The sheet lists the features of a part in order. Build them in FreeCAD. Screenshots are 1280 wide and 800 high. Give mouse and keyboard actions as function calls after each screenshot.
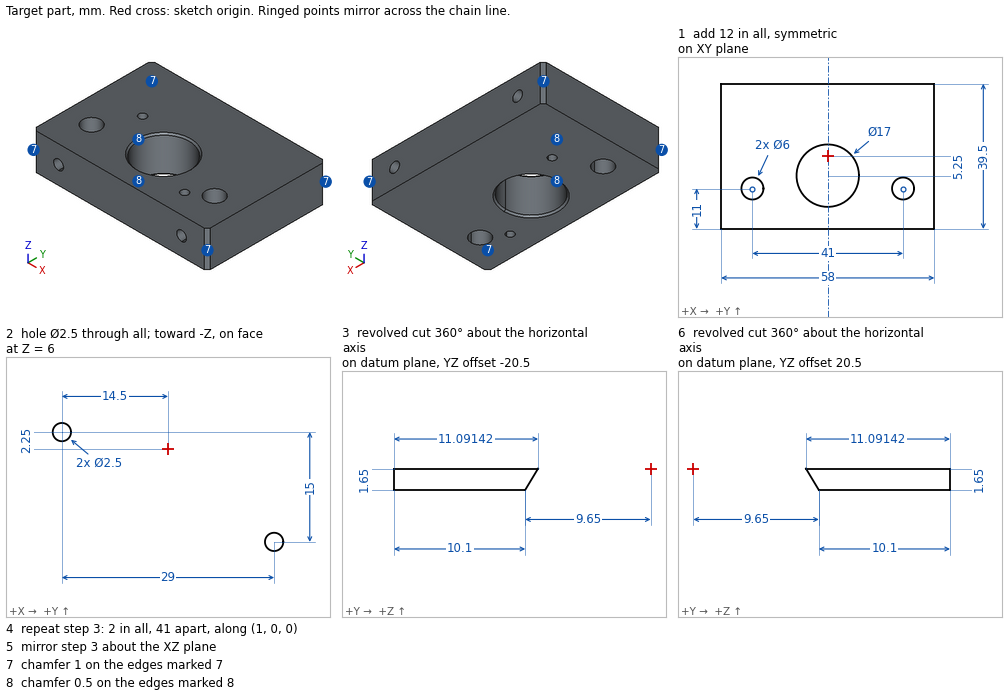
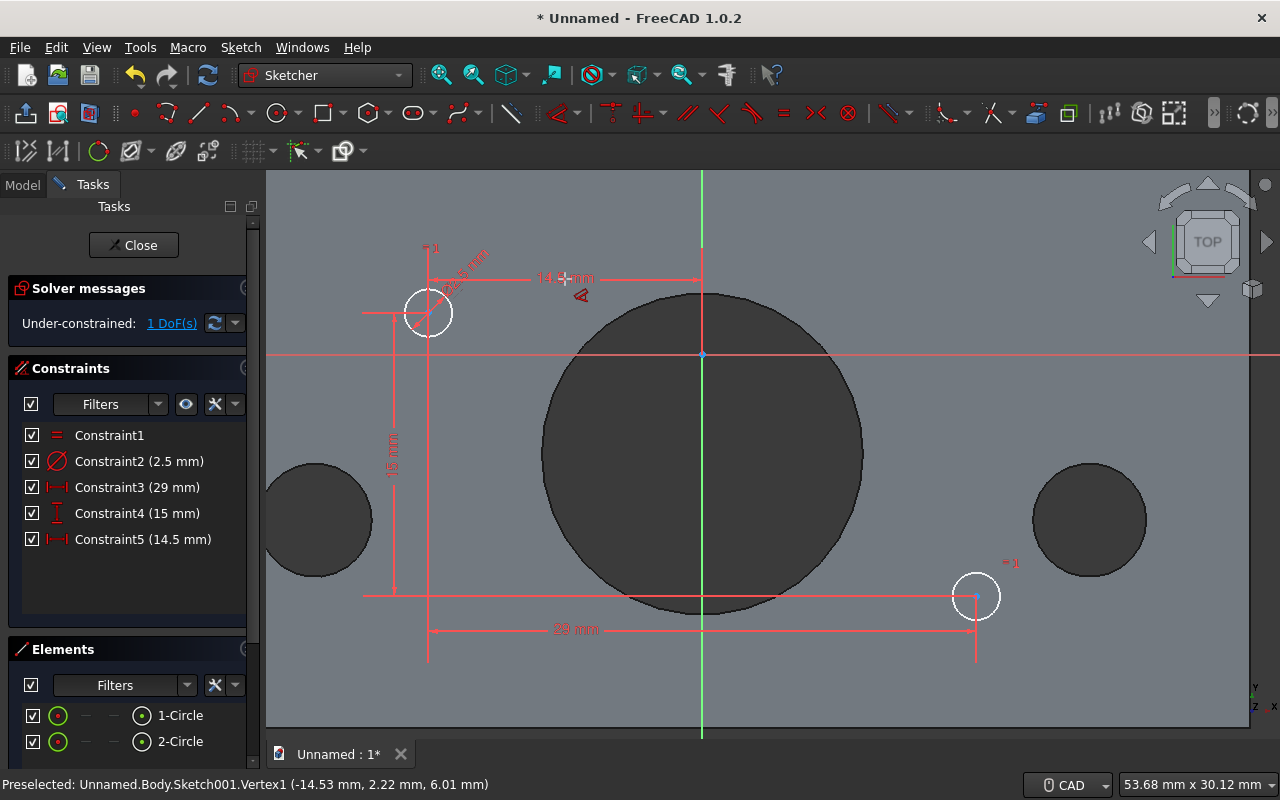
click(428, 313)
click(394, 334)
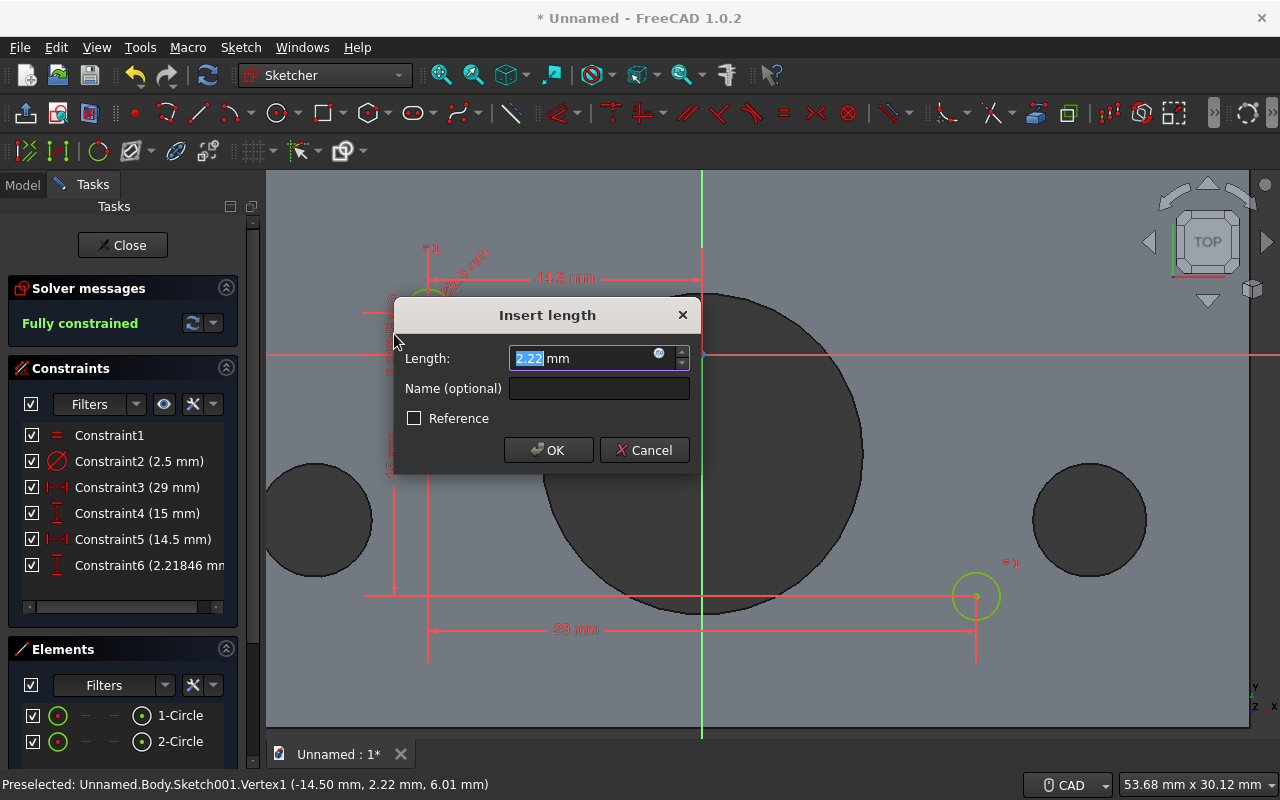
text(2.25)
key(Return)
key(Escape)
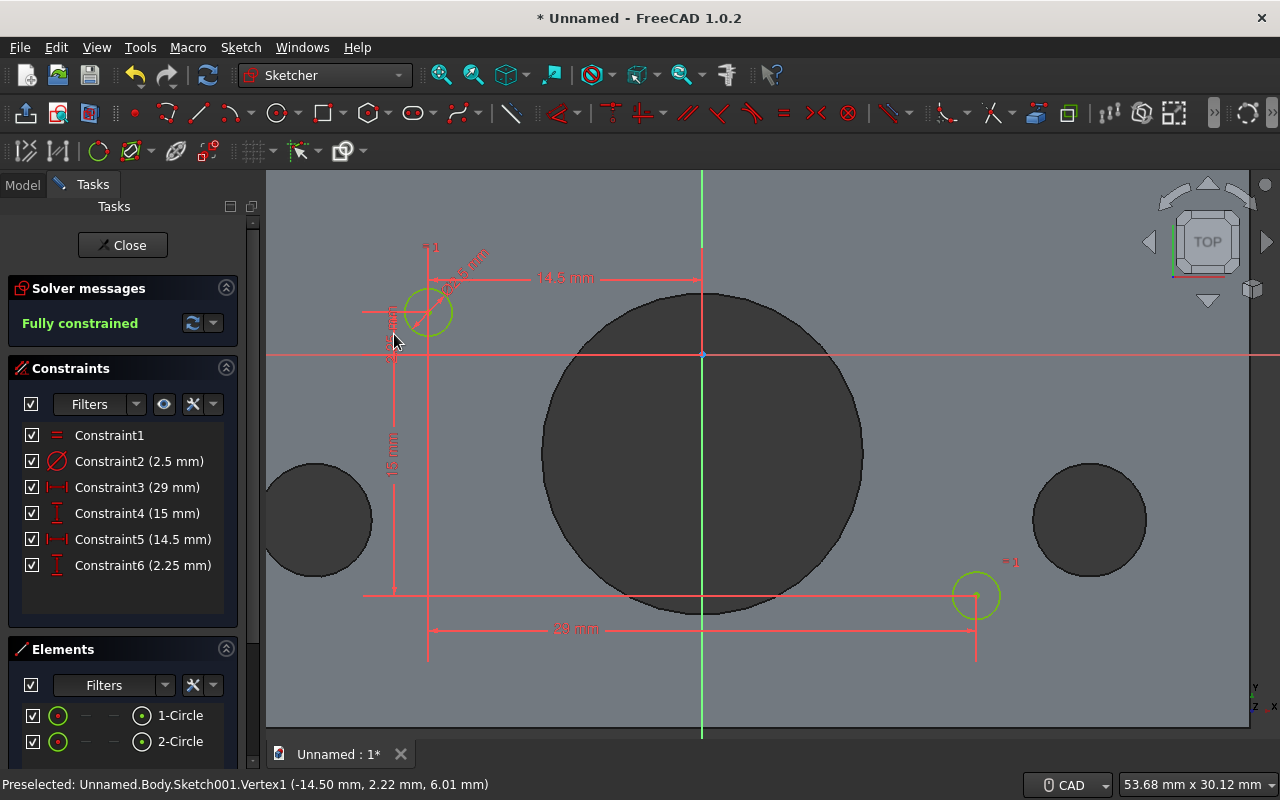
click(123, 245)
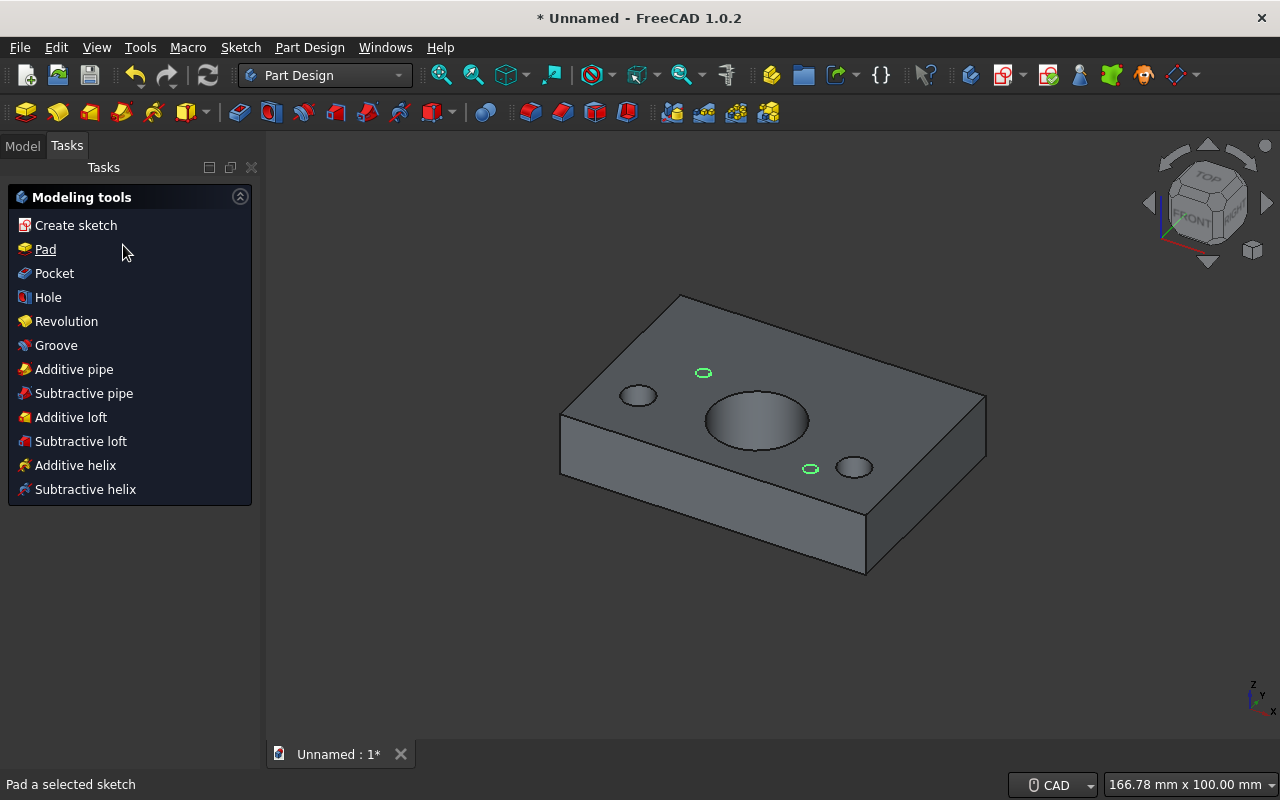
click(272, 112)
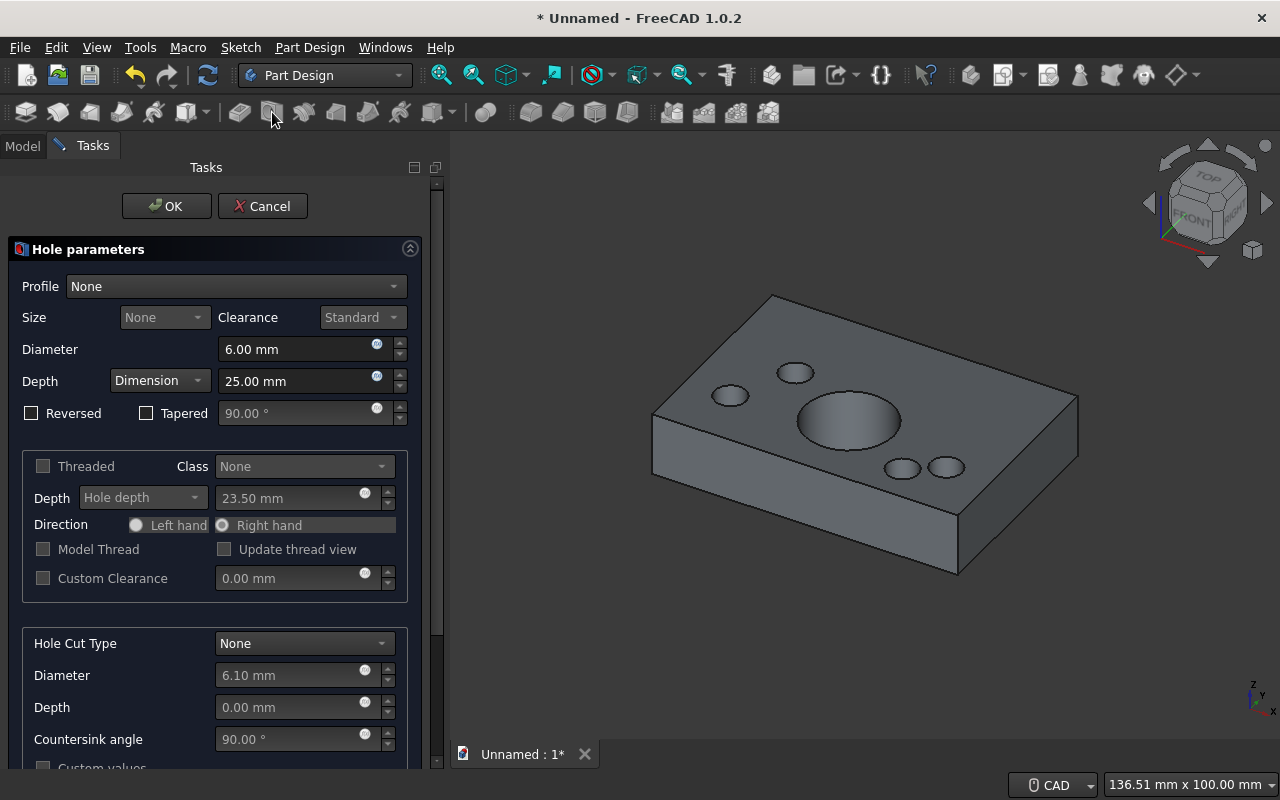
triple_click(305, 349)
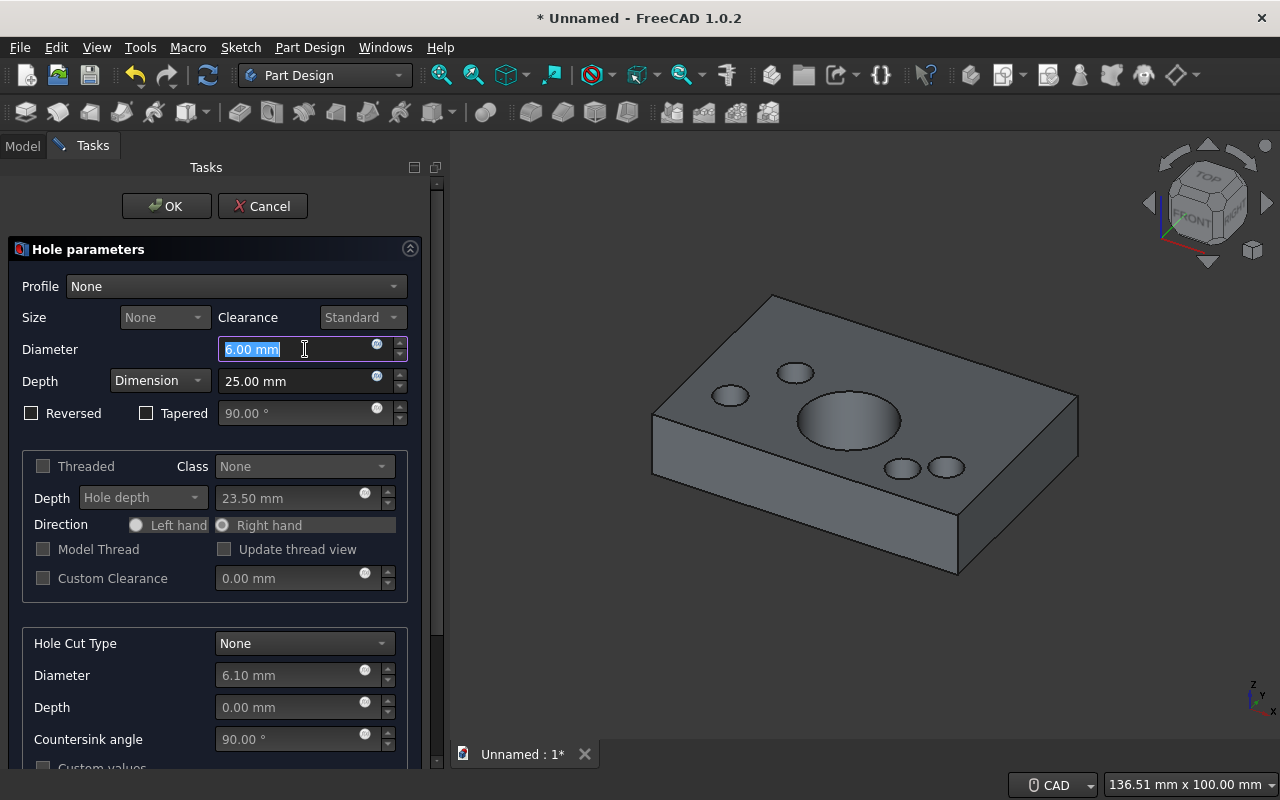
text(2.5)
key(Tab)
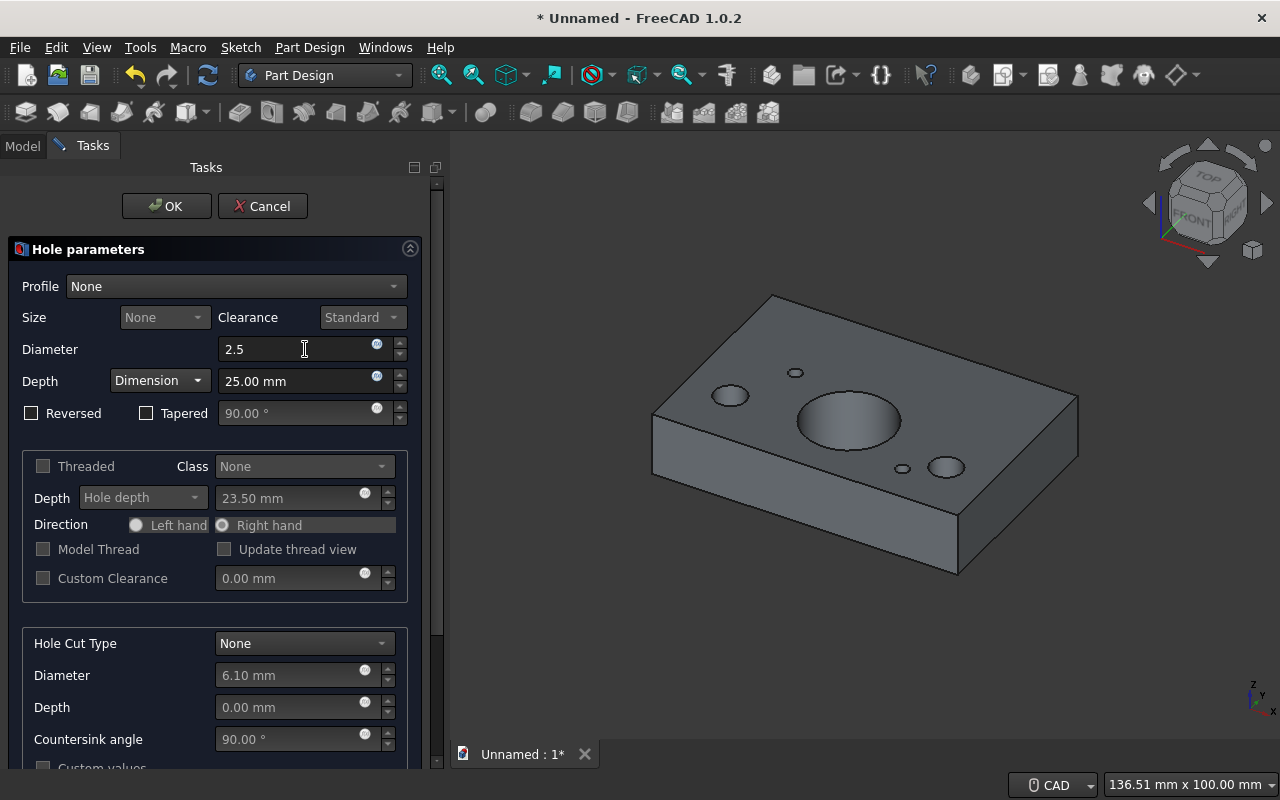
click(161, 380)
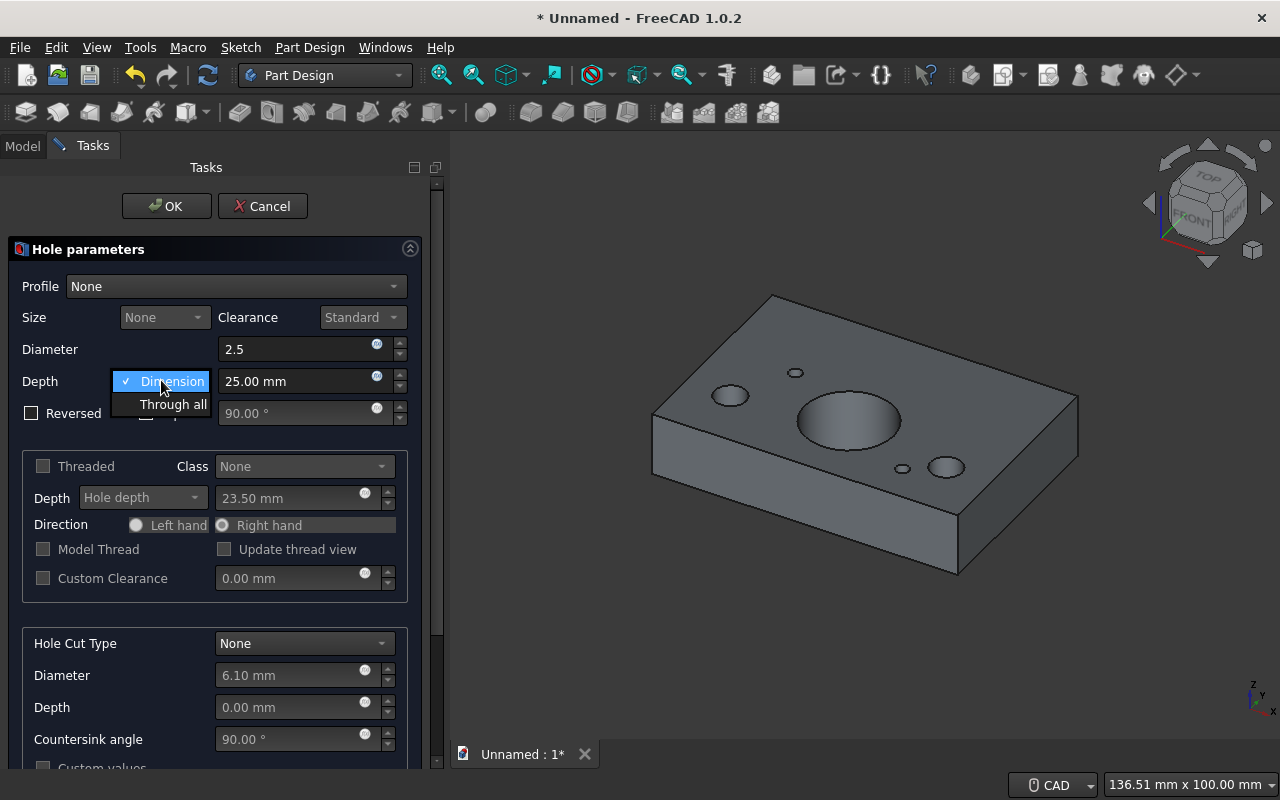
click(160, 404)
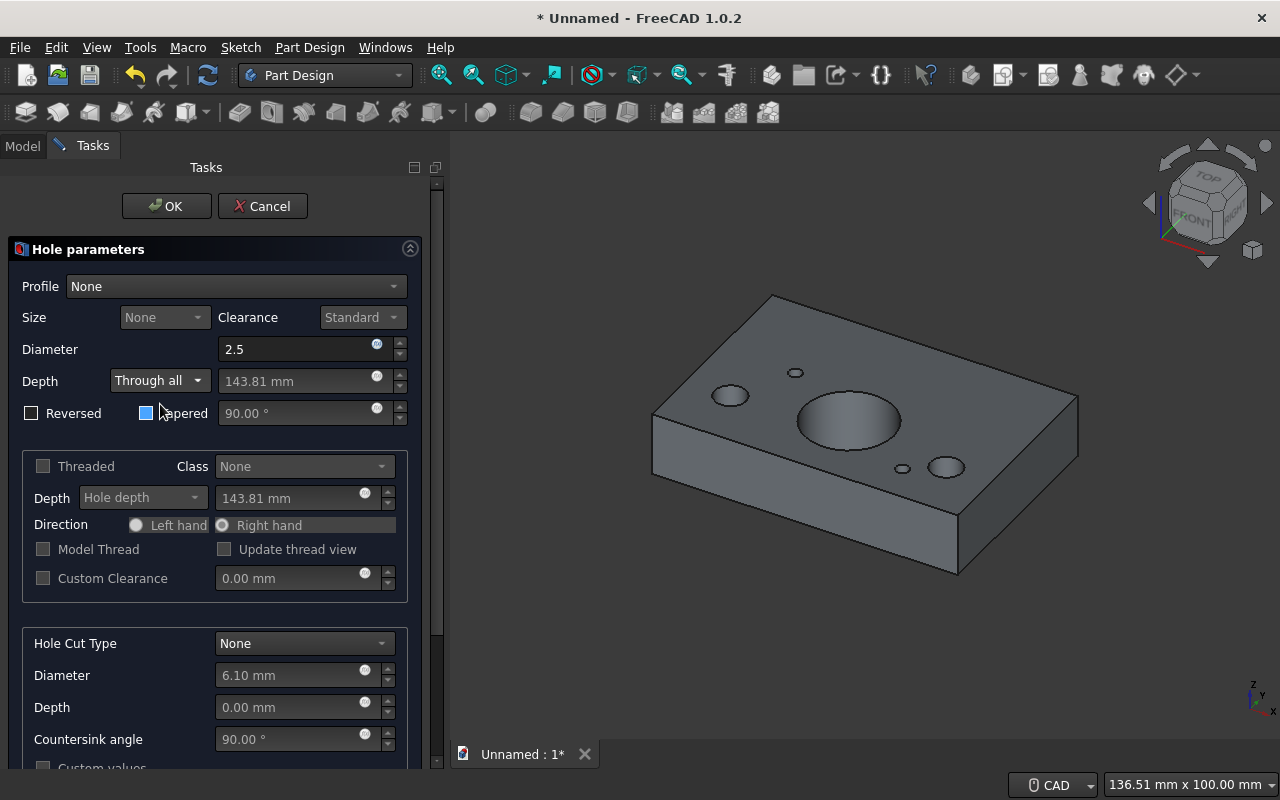
click(167, 206)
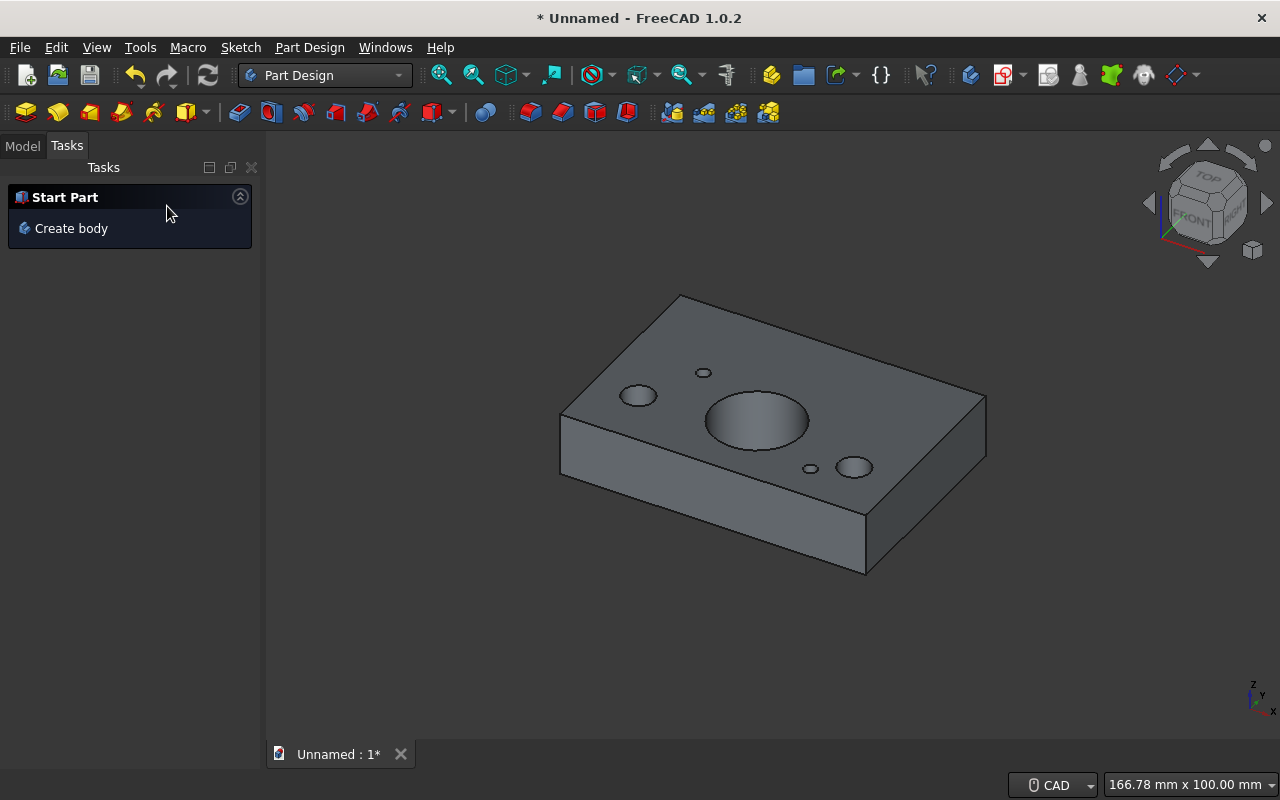
click(23, 145)